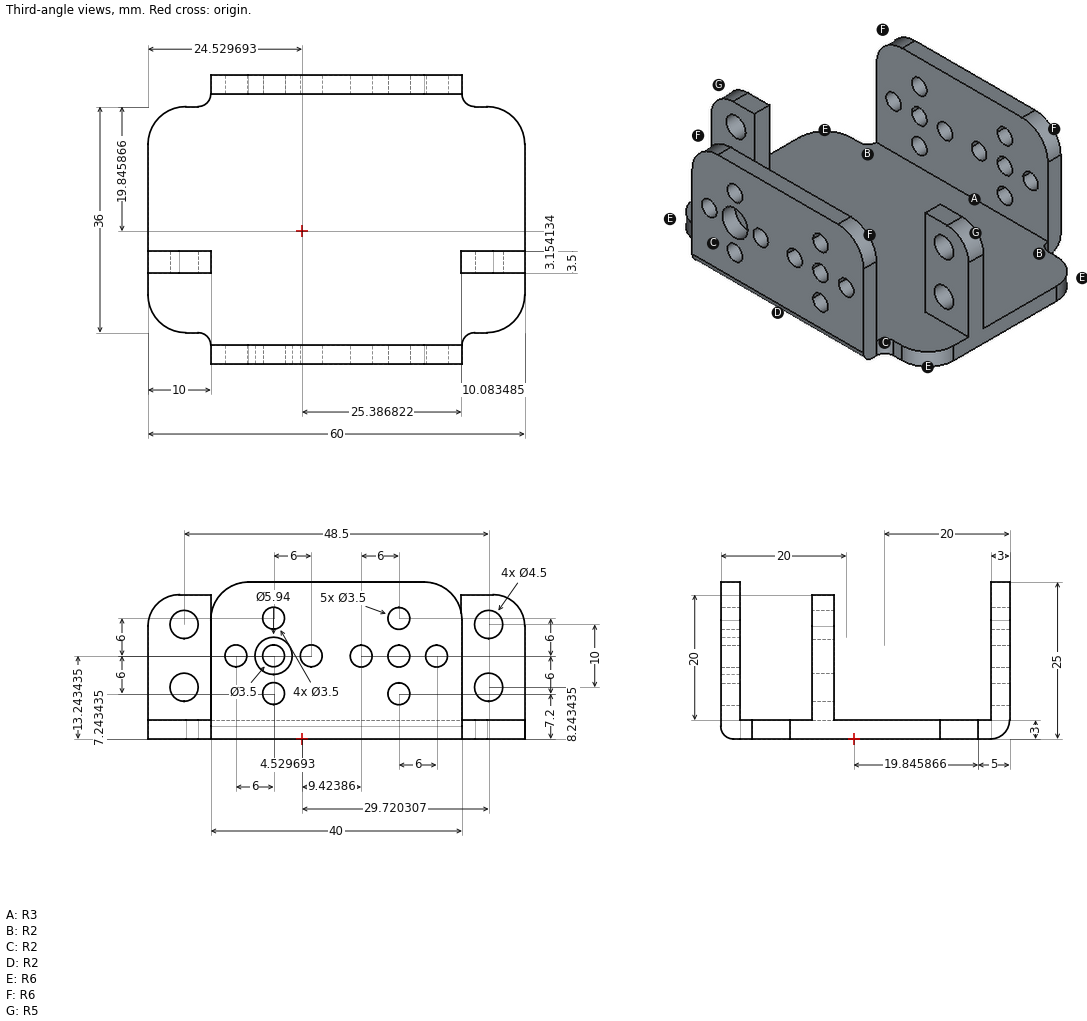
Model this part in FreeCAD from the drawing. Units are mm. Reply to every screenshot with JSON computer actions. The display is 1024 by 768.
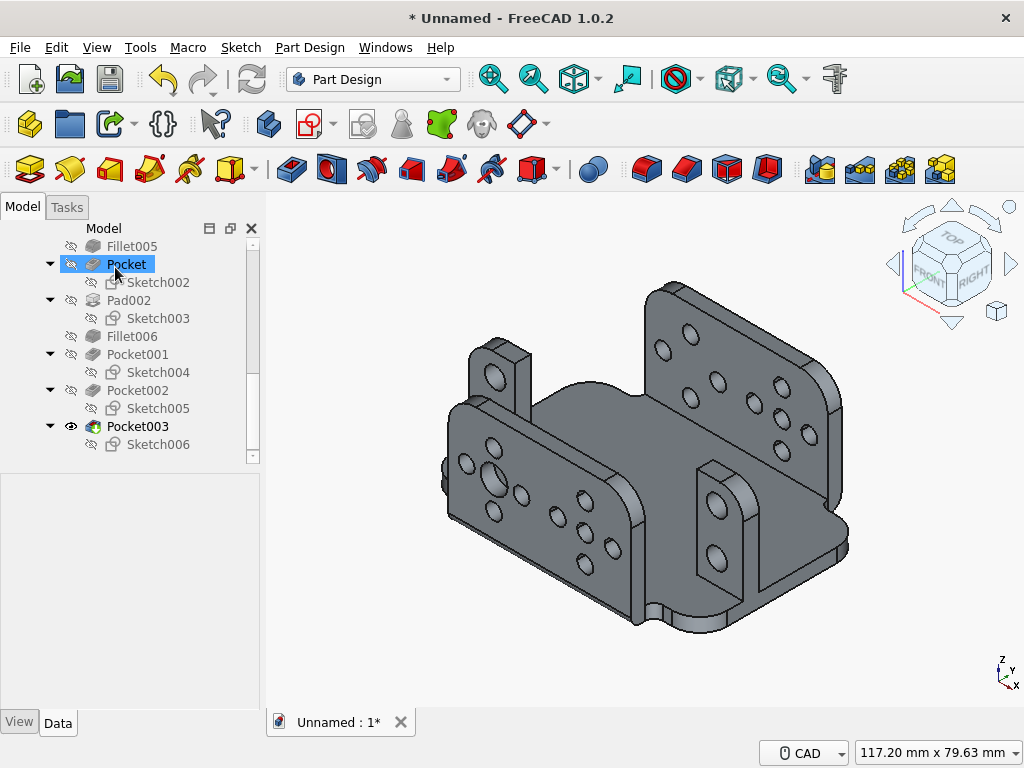
{"action": "key", "text": "4"}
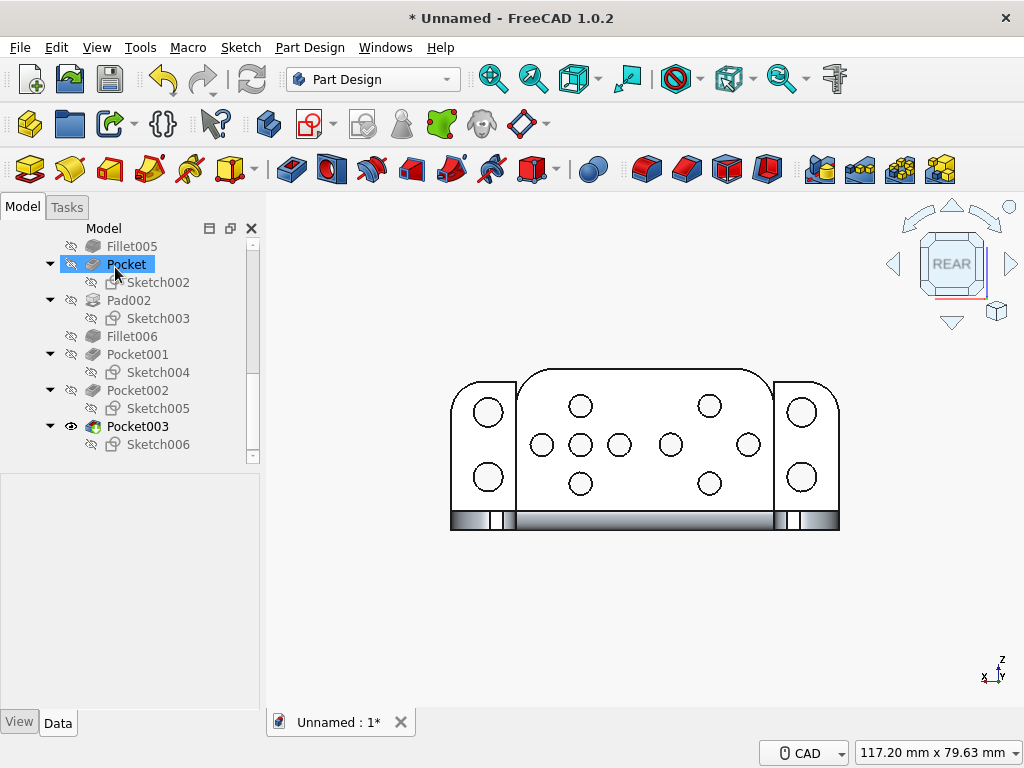
{"action": "left_click", "coordinate": [645, 398]}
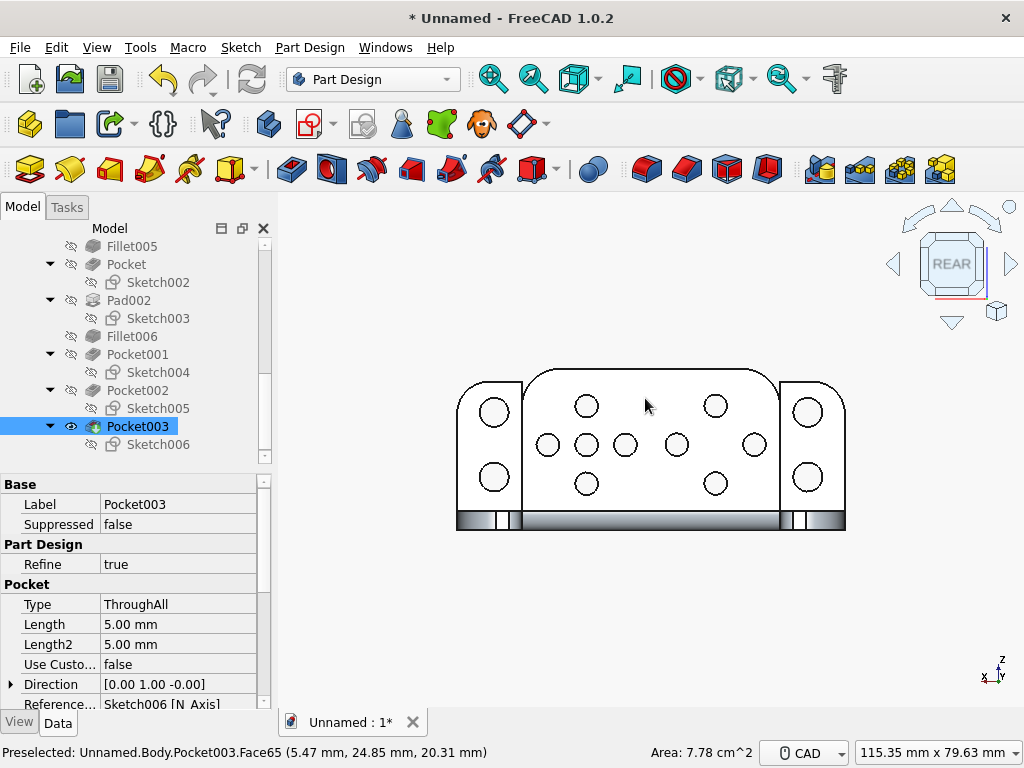
{"action": "left_click", "coordinate": [310, 124]}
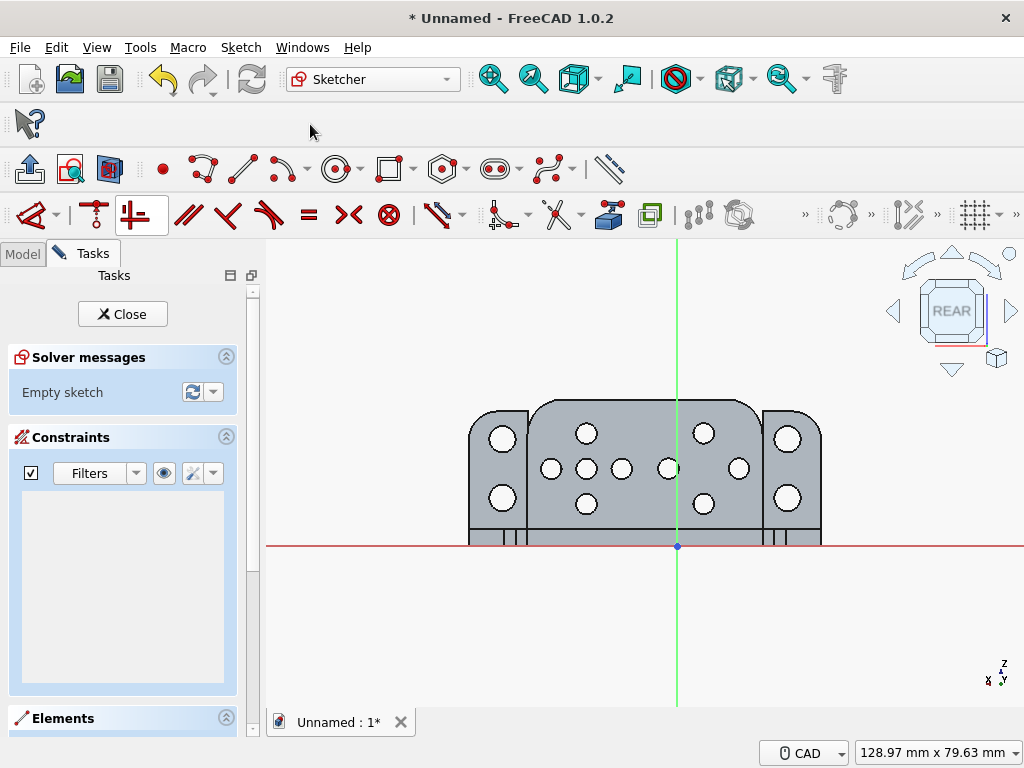
{"action": "scroll", "coordinate": [714, 468], "scroll_direction": "up", "scroll_amount": 13}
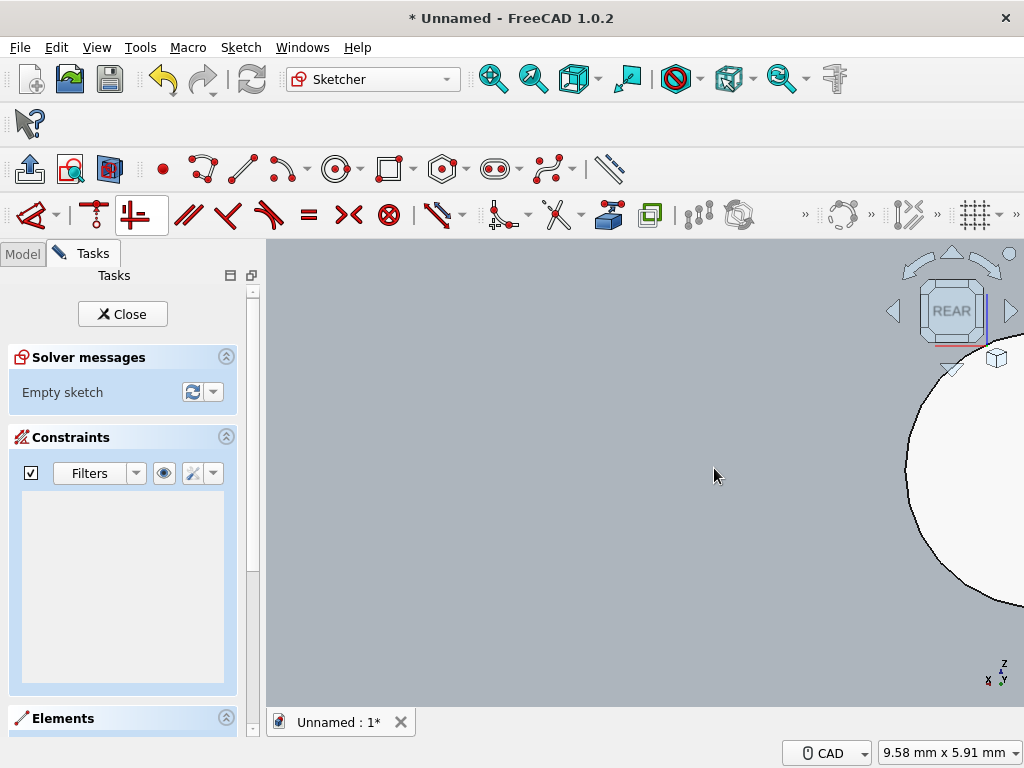
{"action": "left_click", "coordinate": [336, 170]}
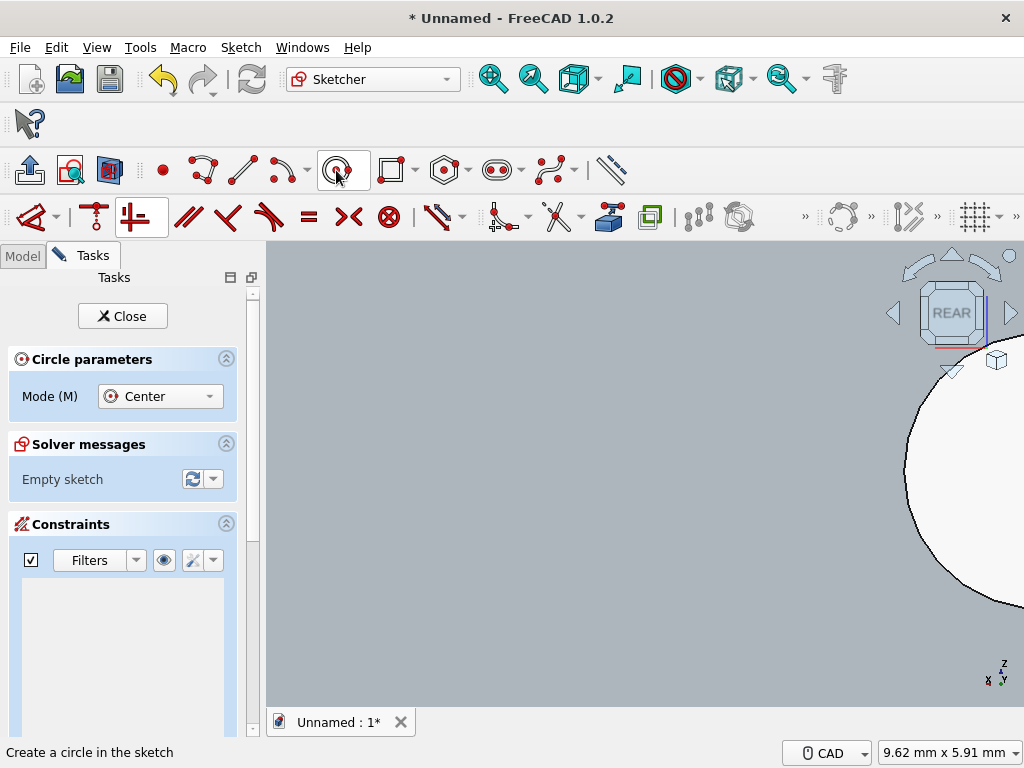
{"action": "left_click", "coordinate": [569, 471]}
{"action": "left_click", "coordinate": [667, 374]}
{"action": "key", "text": "Escape"}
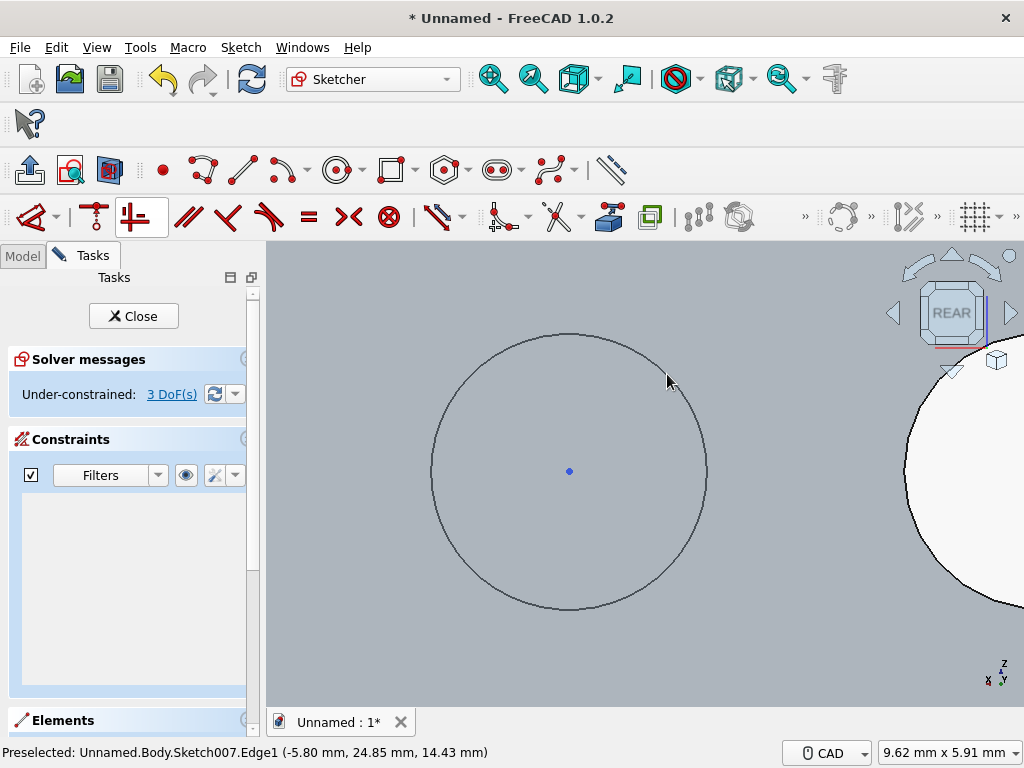
{"action": "left_click", "coordinate": [32, 218]}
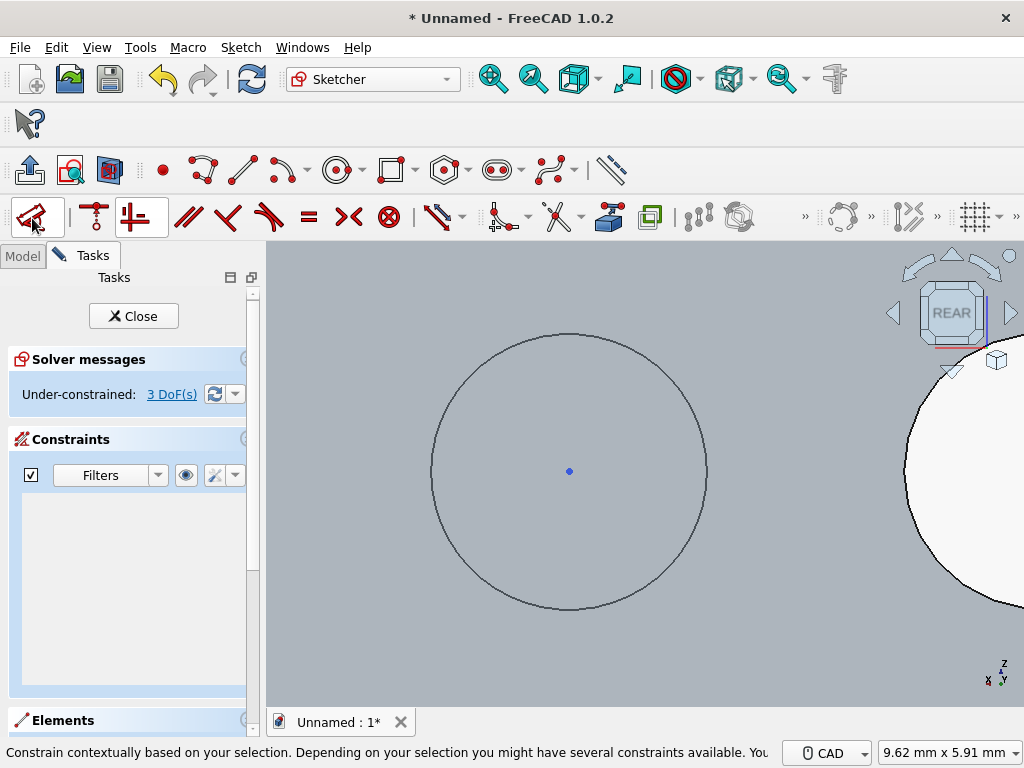
{"action": "left_click", "coordinate": [666, 374]}
{"action": "left_click", "coordinate": [689, 351]}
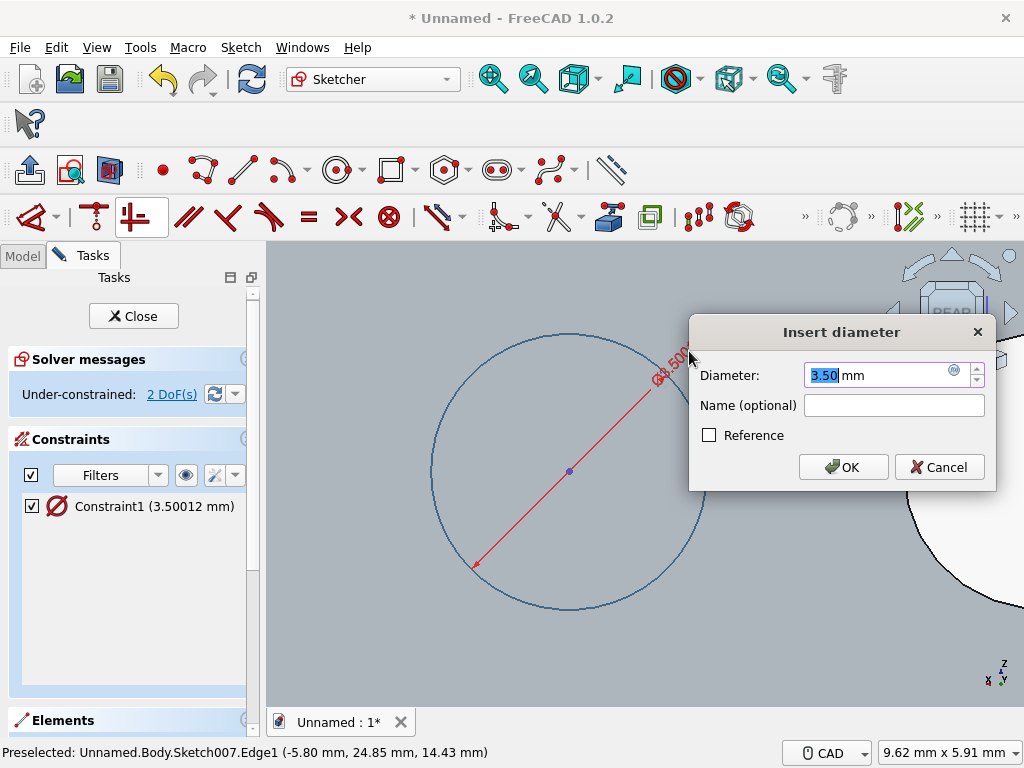
{"action": "type", "text": "3.5"}
{"action": "key", "text": "Return"}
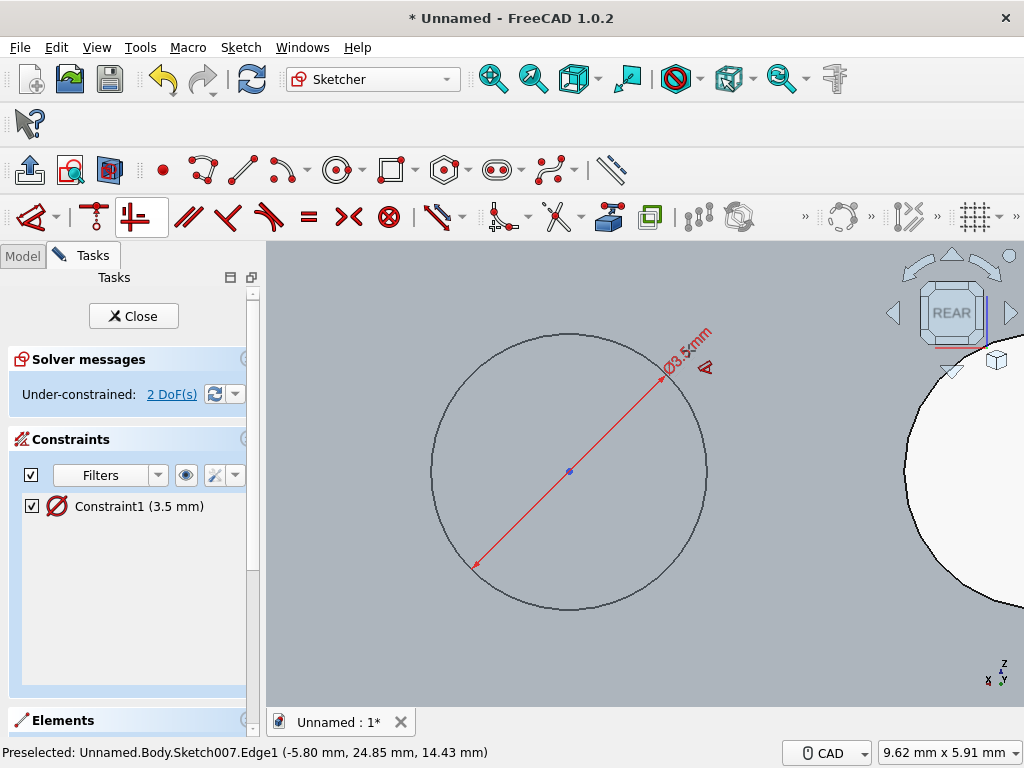
{"action": "left_click", "coordinate": [569, 472]}
{"action": "left_click", "coordinate": [368, 438]}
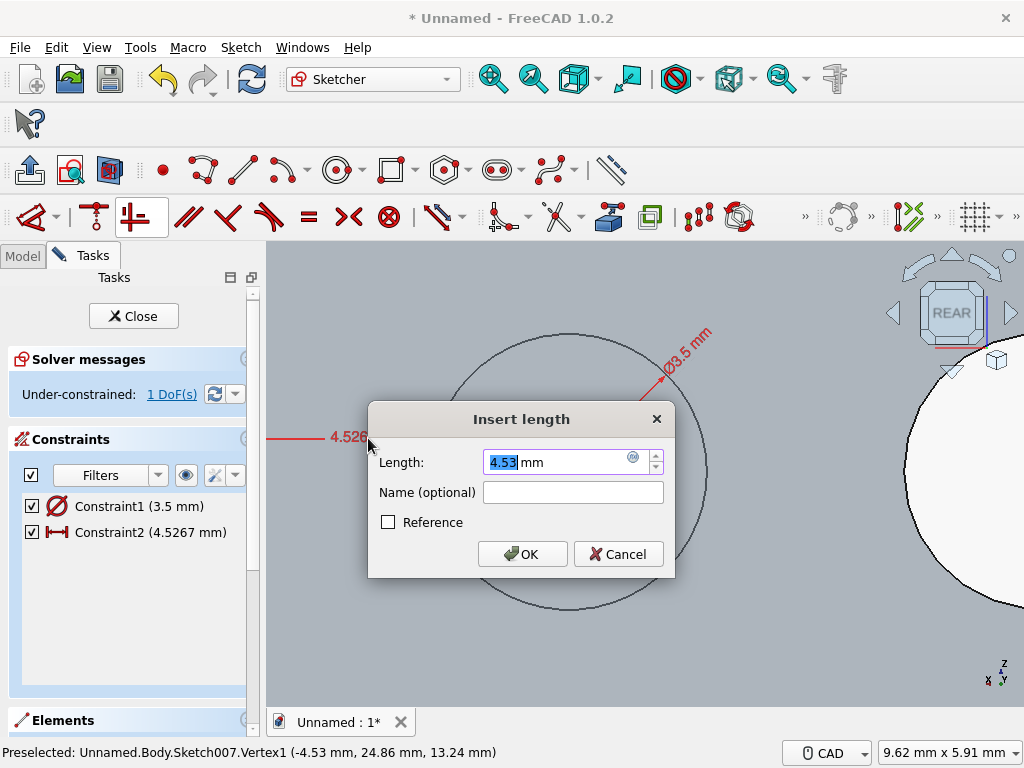
{"action": "type", "text": "4.529693"}
{"action": "key", "text": "Return"}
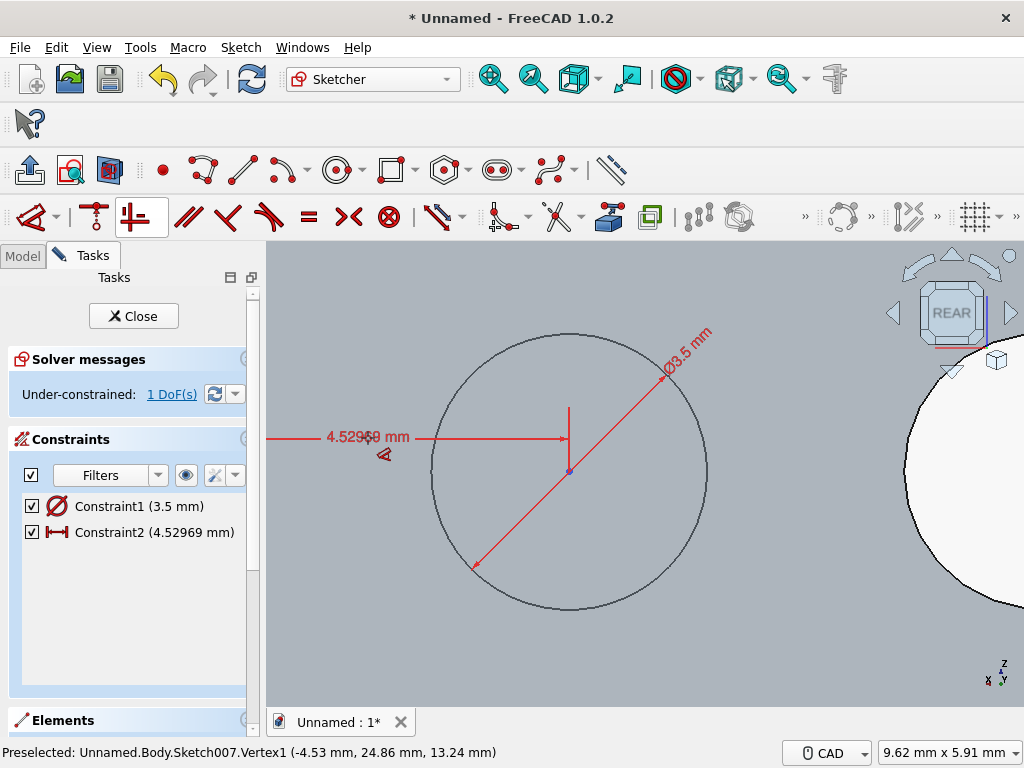
{"action": "left_click", "coordinate": [569, 472]}
{"action": "left_click", "coordinate": [603, 575]}